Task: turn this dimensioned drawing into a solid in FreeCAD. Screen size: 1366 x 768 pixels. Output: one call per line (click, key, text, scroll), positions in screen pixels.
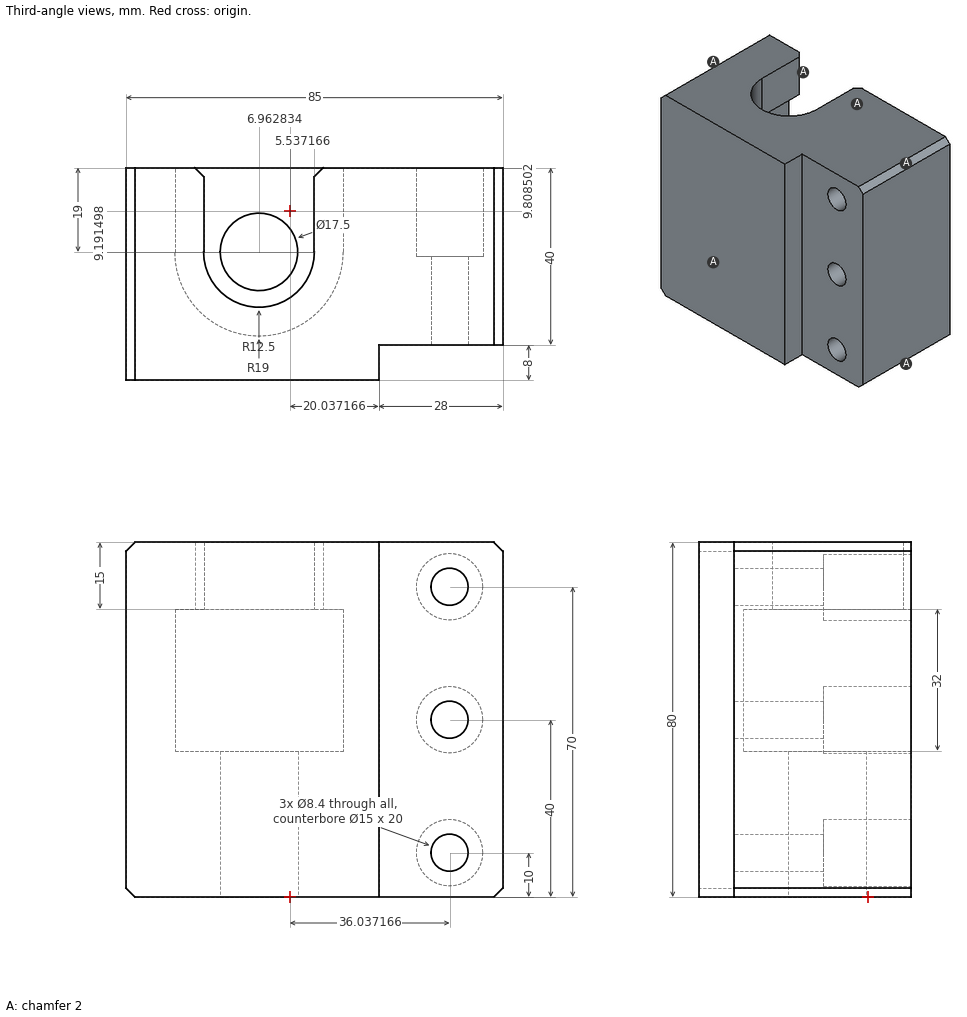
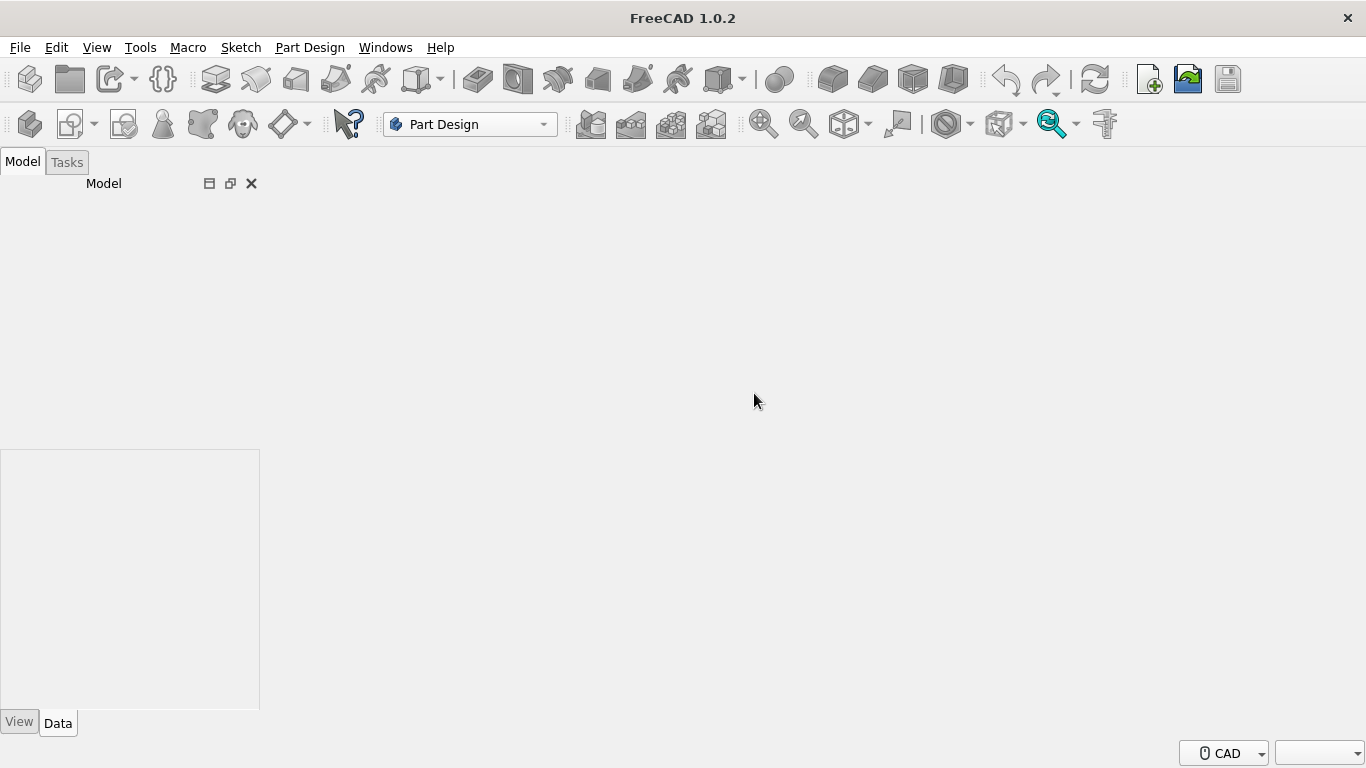
key(ctrl+n)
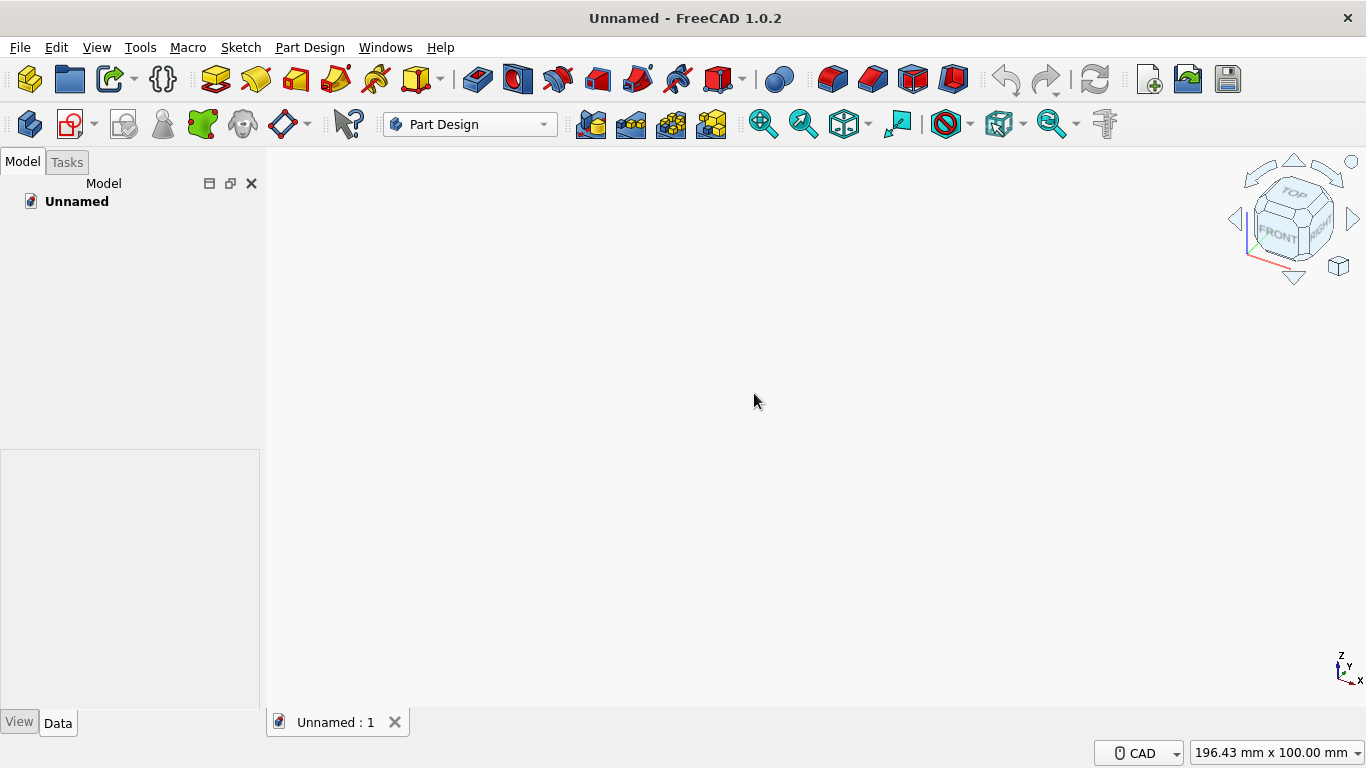
click(70, 124)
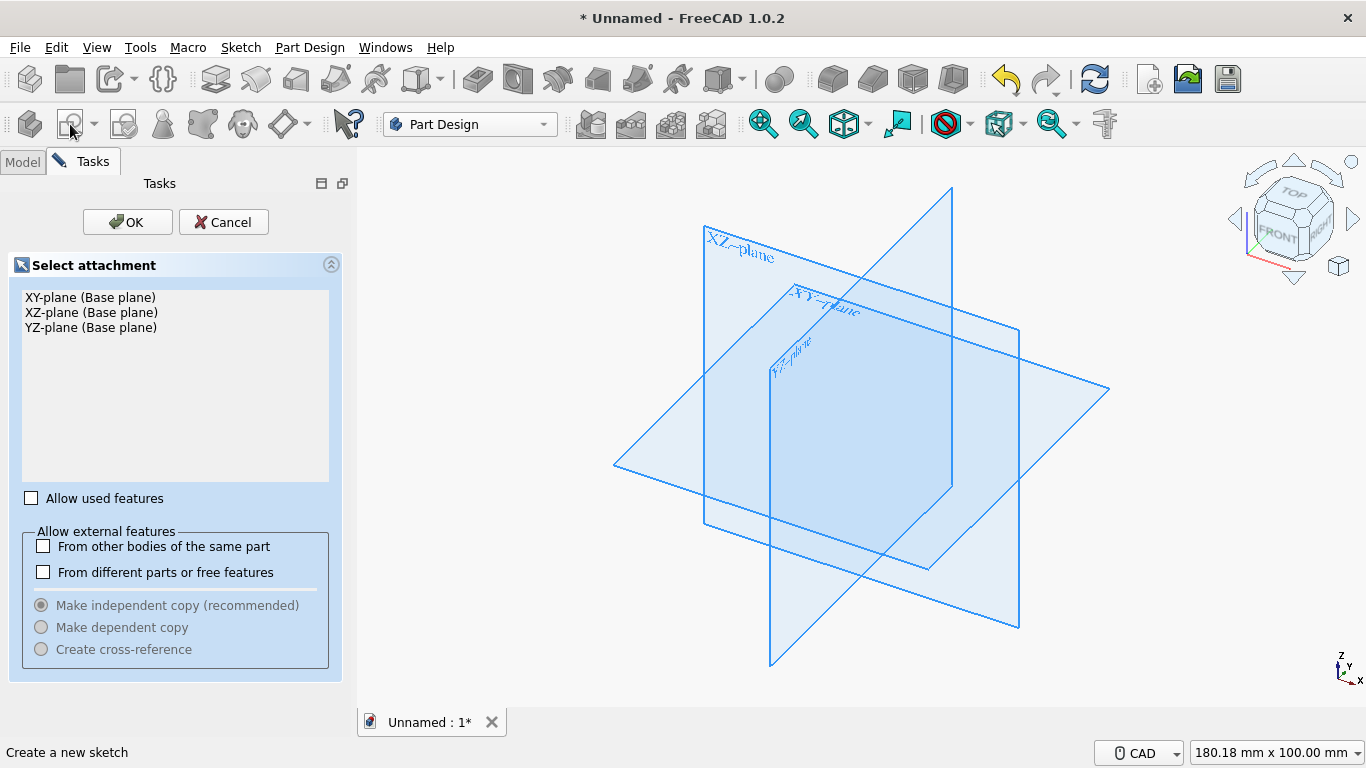
click(82, 298)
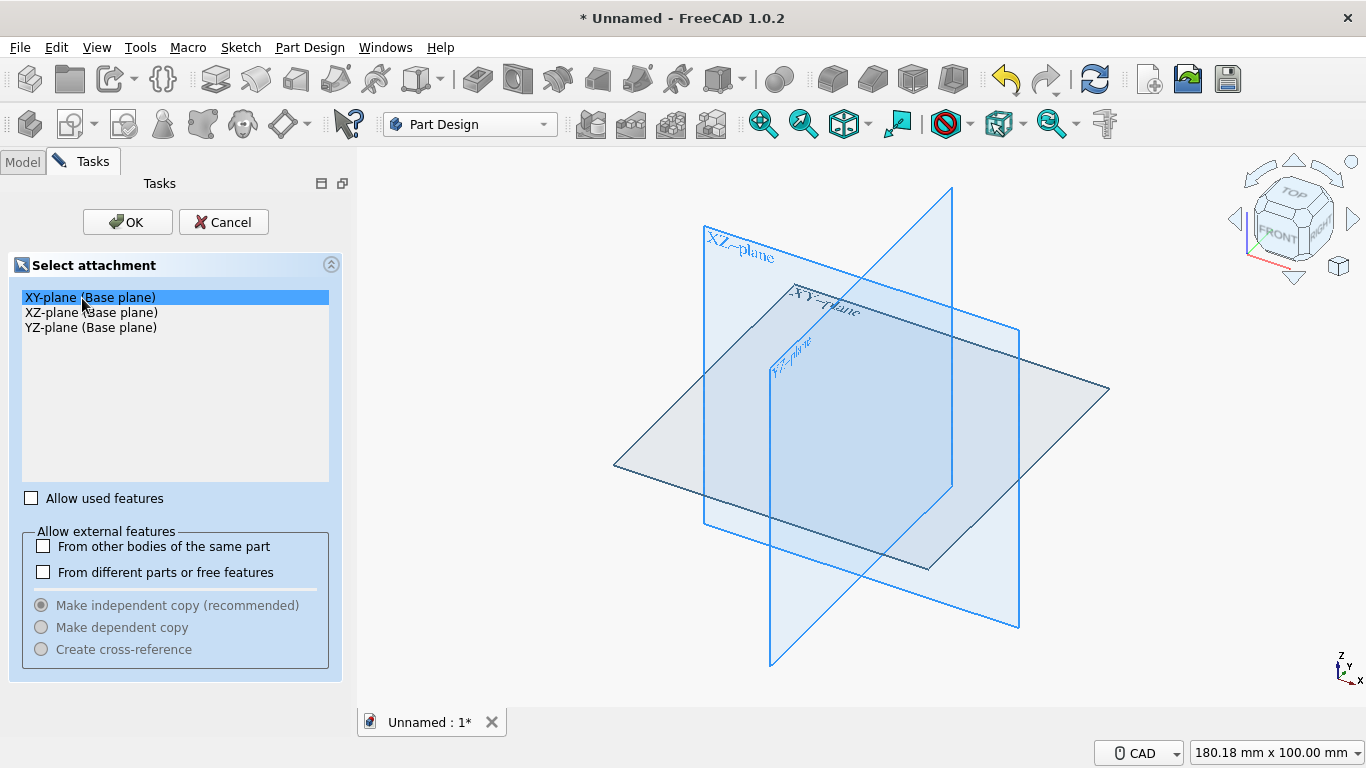
click(128, 222)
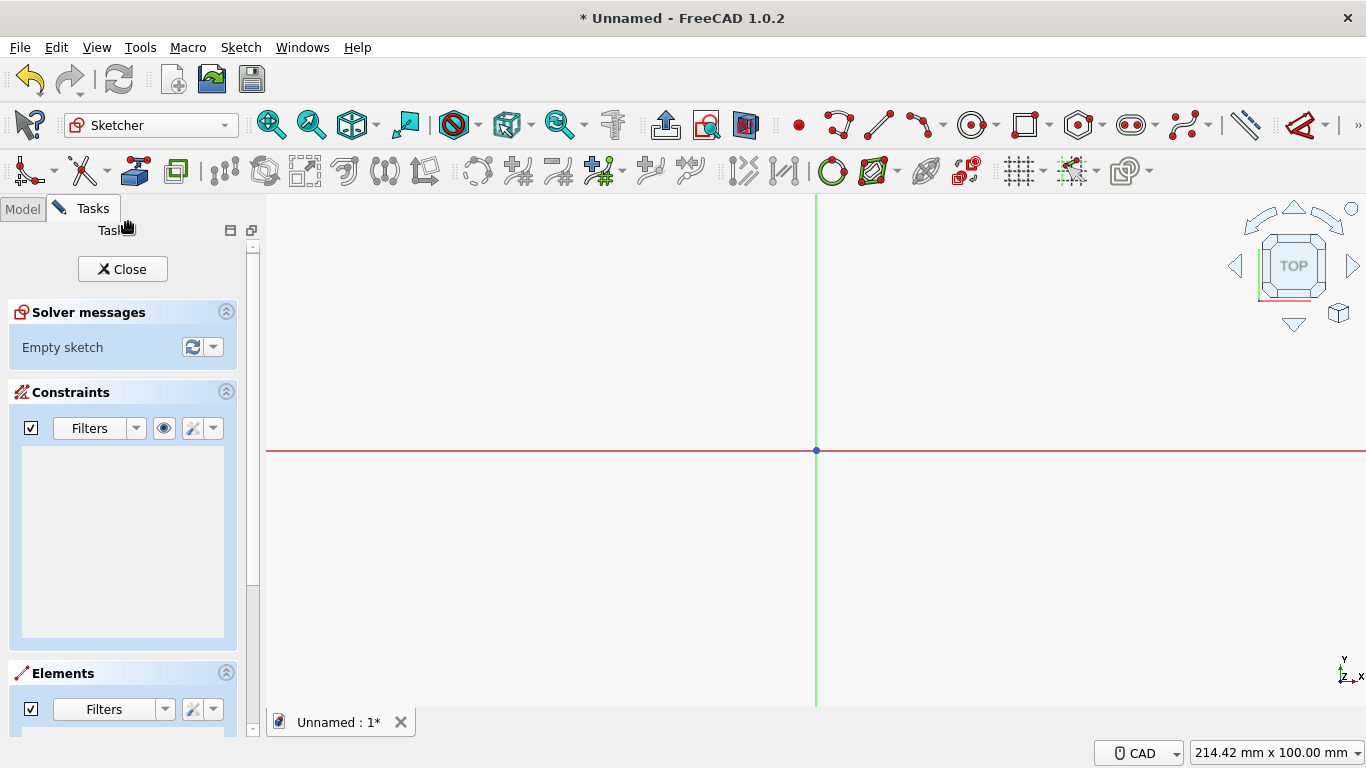
click(840, 126)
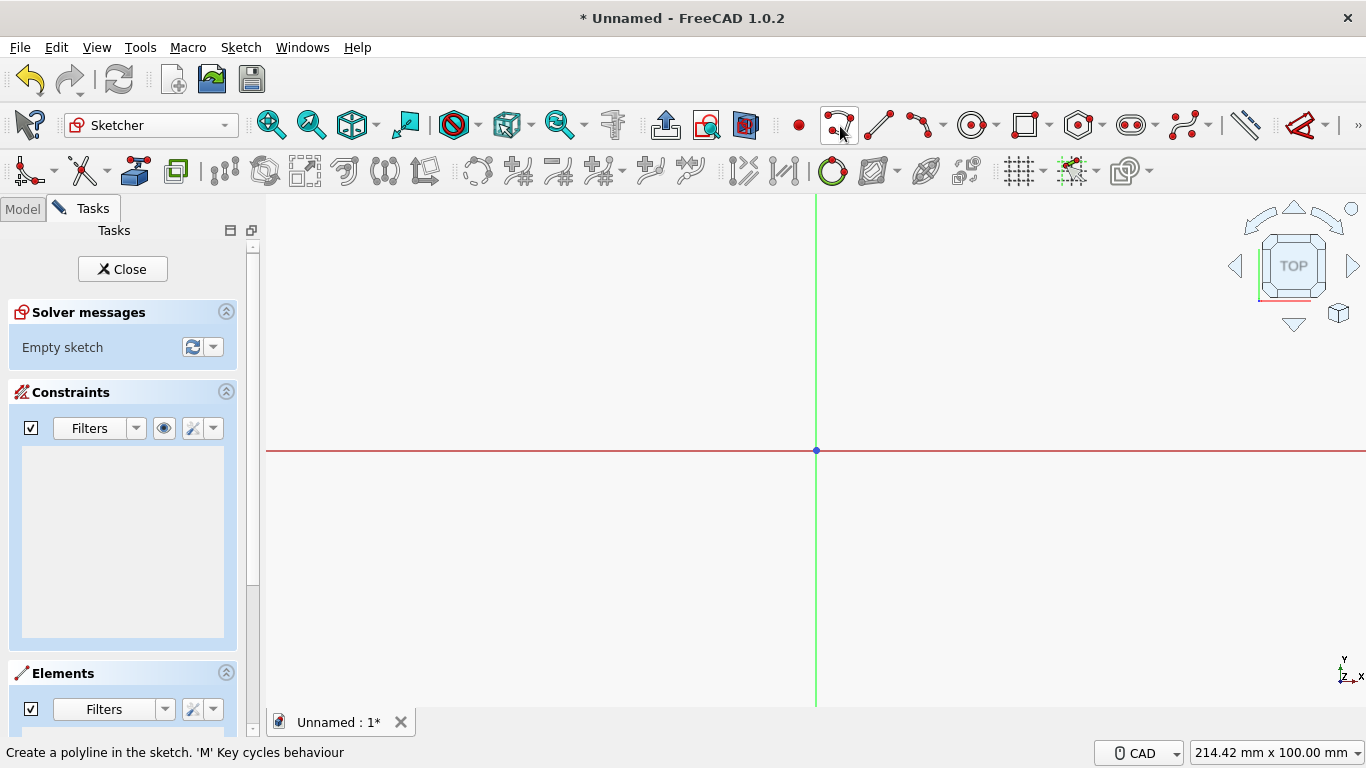
click(919, 605)
click(1062, 605)
click(1062, 400)
click(626, 400)
click(626, 646)
click(919, 646)
click(919, 606)
key(Escape)
key(Escape)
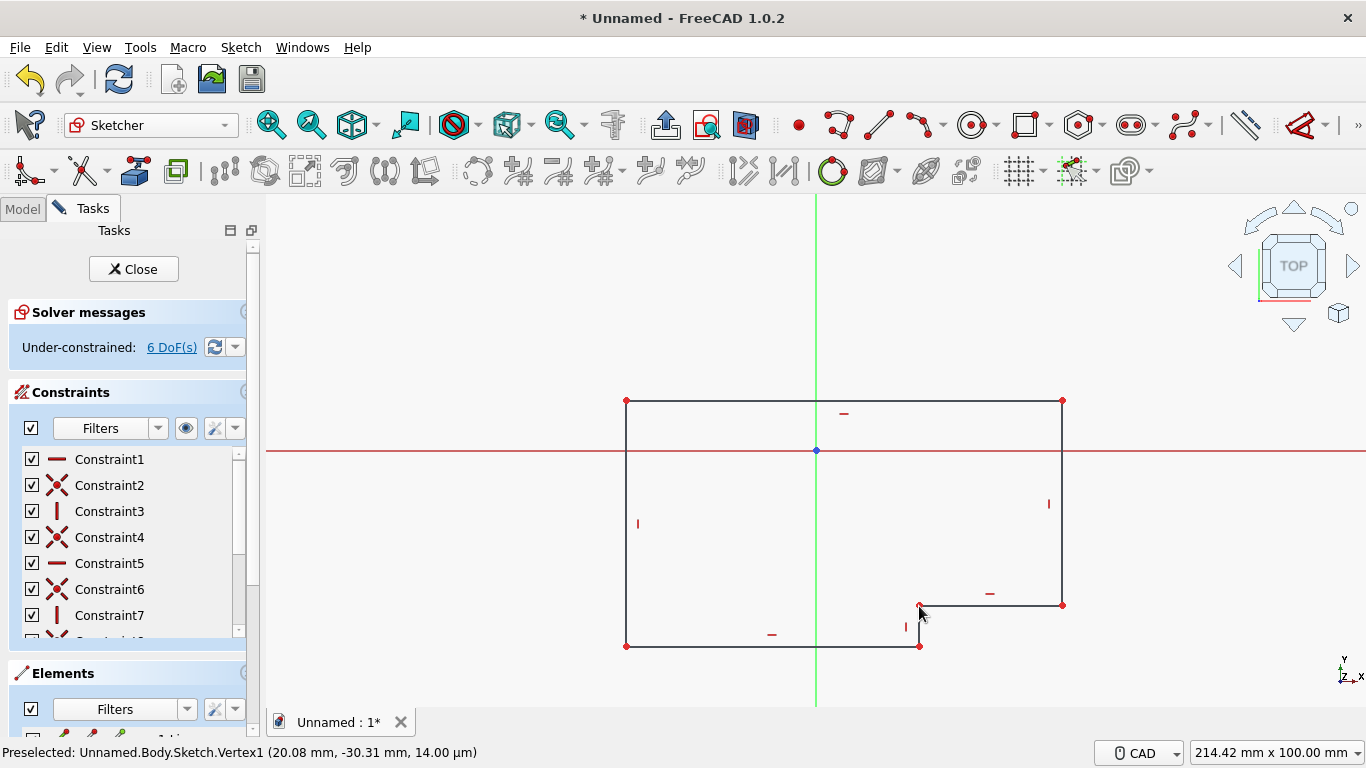
click(1300, 126)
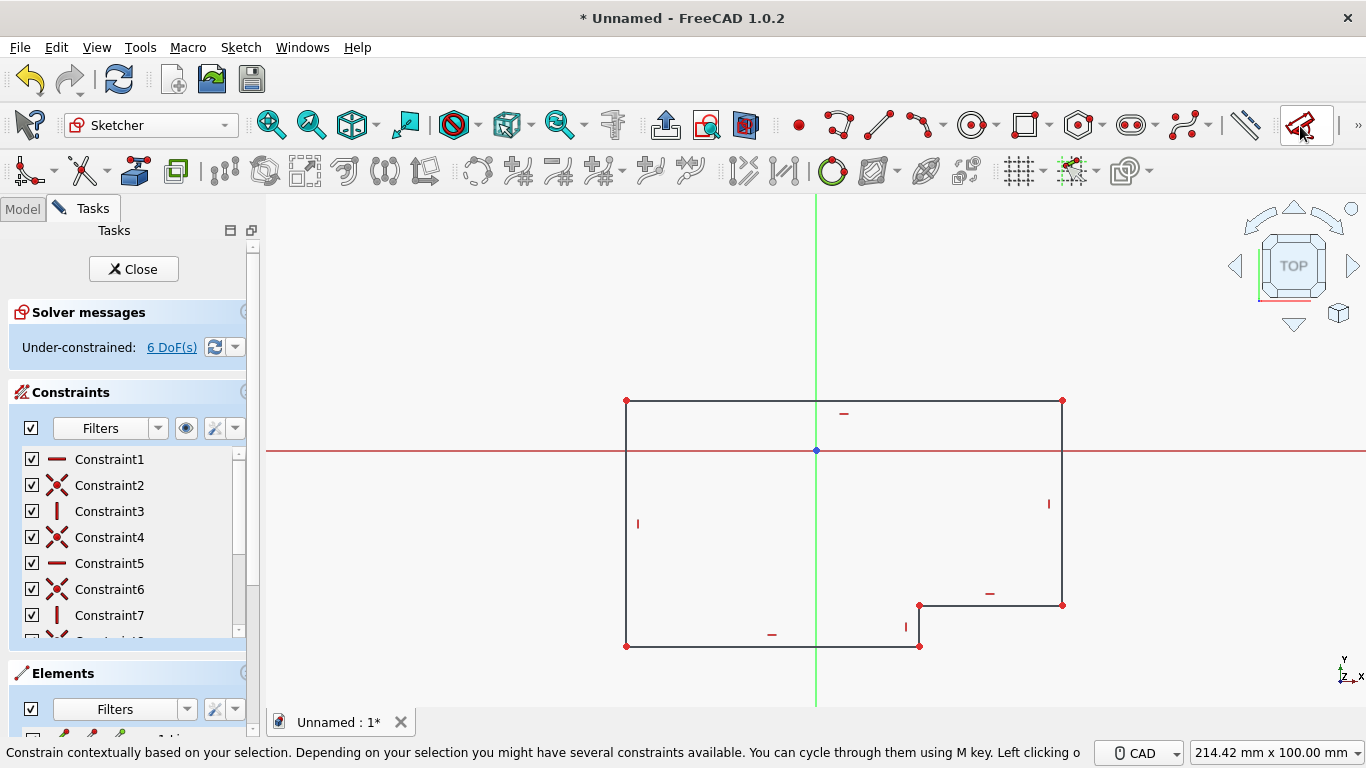
click(919, 635)
click(953, 626)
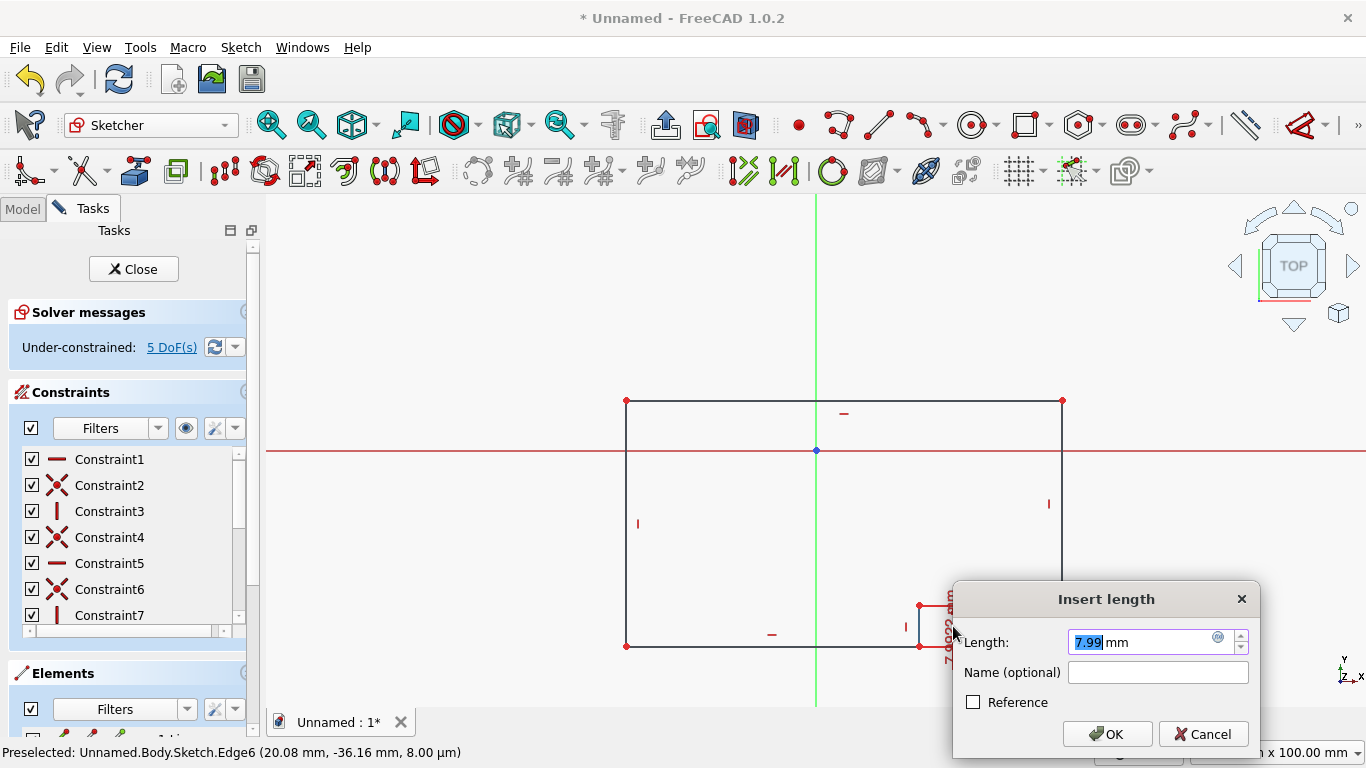
text(8)
key(Return)